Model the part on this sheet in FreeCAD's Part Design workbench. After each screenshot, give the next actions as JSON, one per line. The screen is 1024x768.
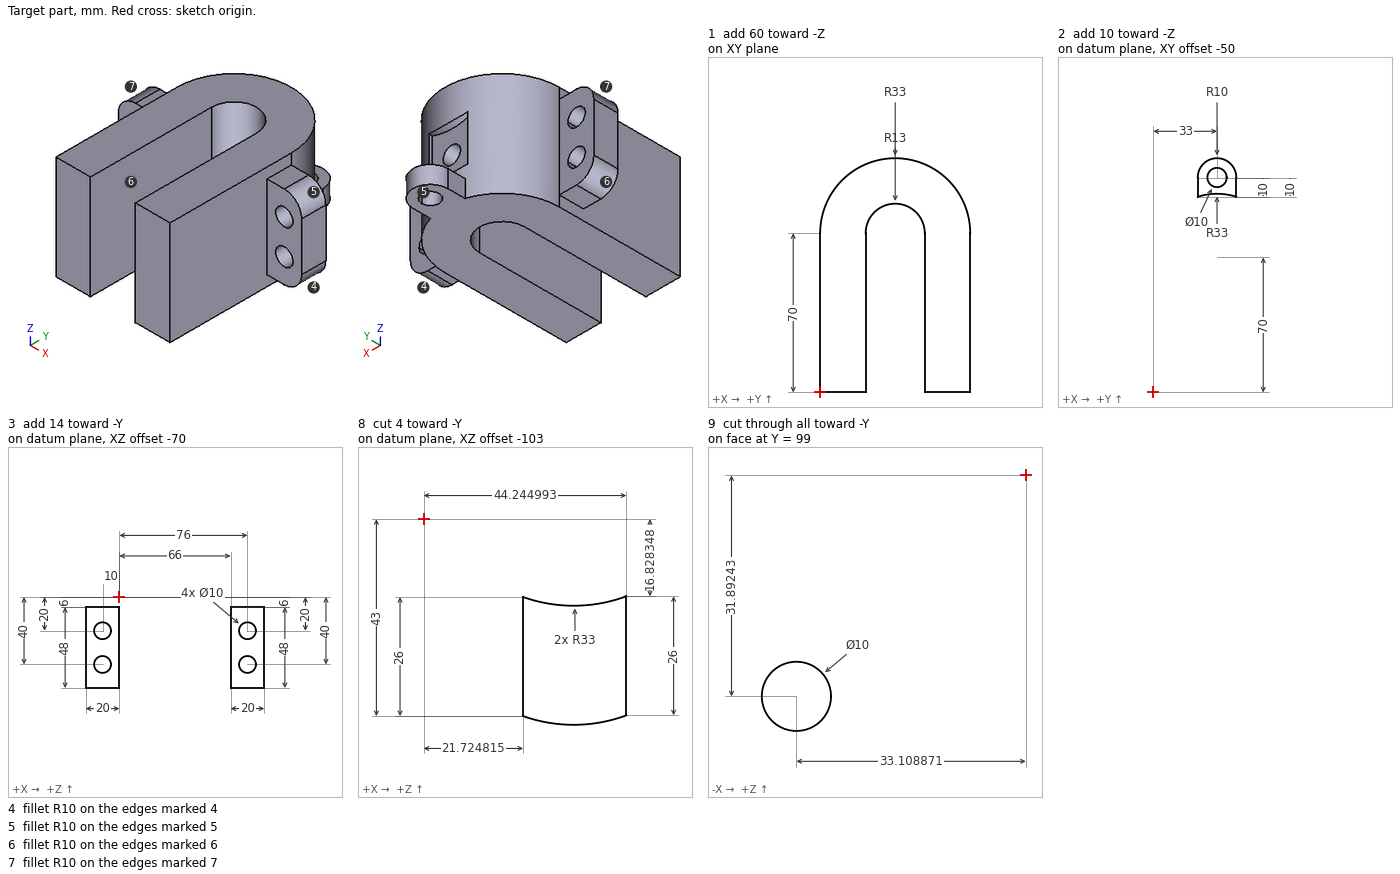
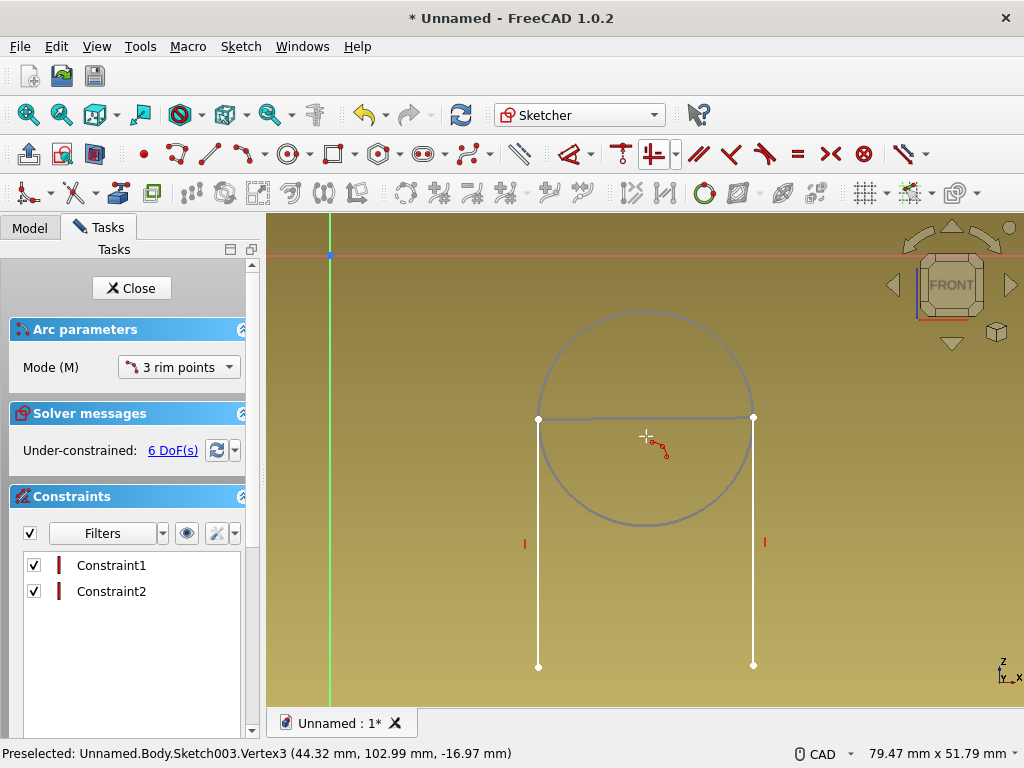
{"action": "left_click", "coordinate": [645, 436]}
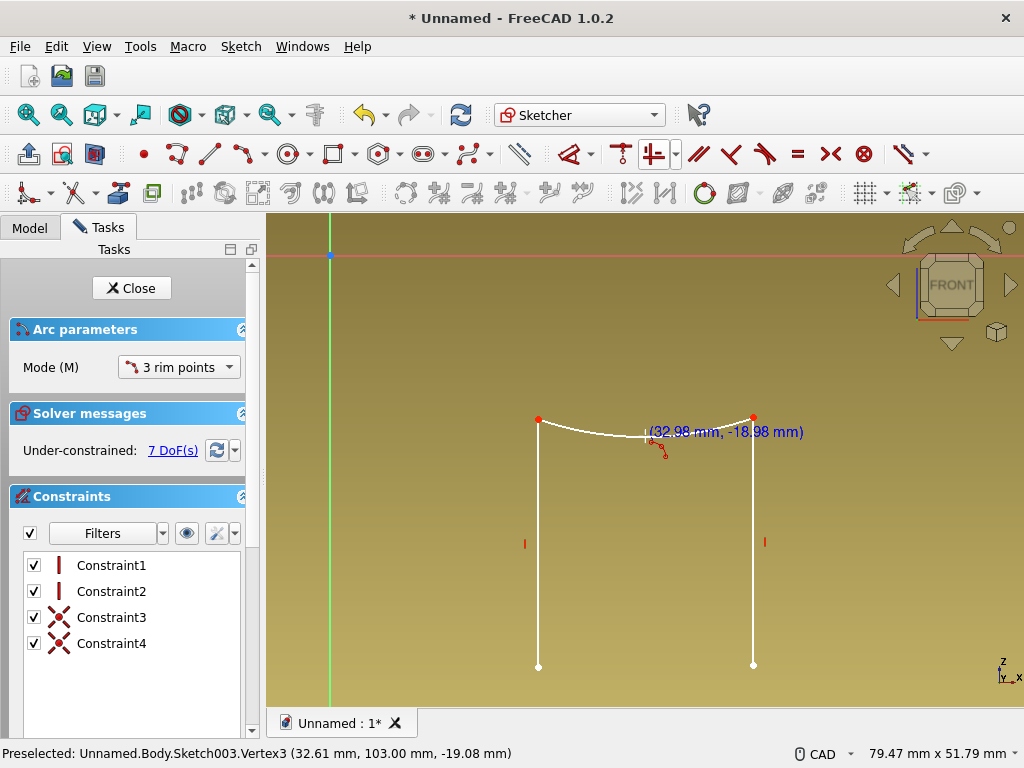
{"action": "left_click", "coordinate": [753, 666]}
{"action": "left_click", "coordinate": [538, 667]}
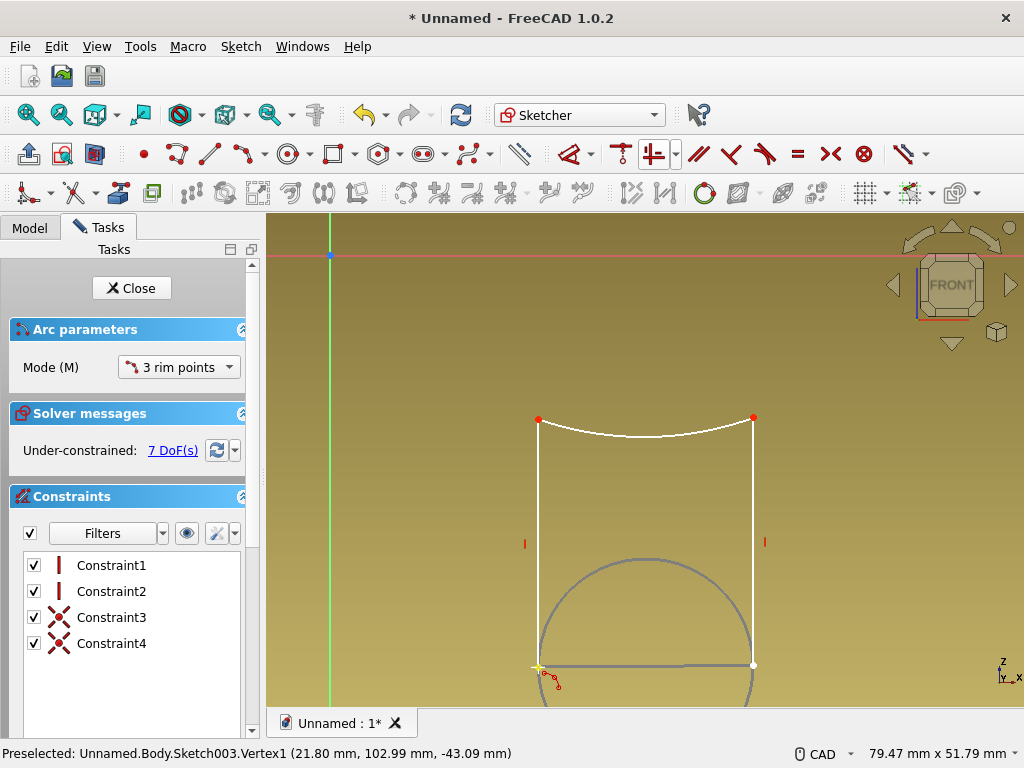
{"action": "scroll", "coordinate": [648, 440], "scroll_direction": "down", "scroll_amount": 2}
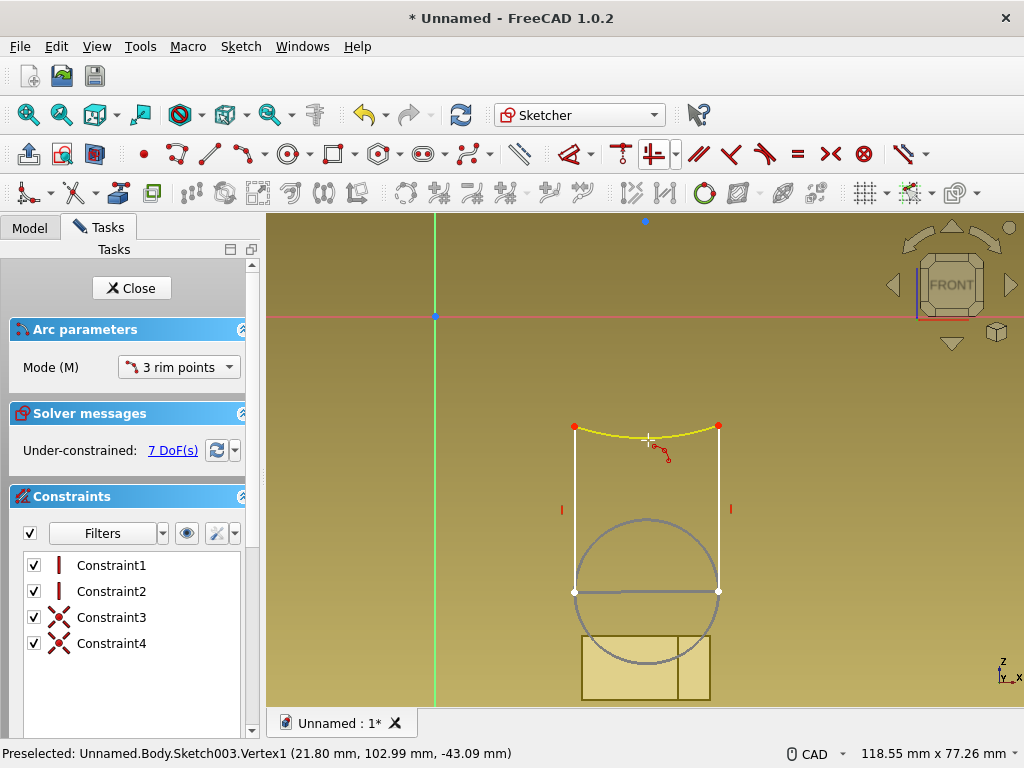
{"action": "scroll", "coordinate": [646, 604], "scroll_direction": "up", "scroll_amount": 2}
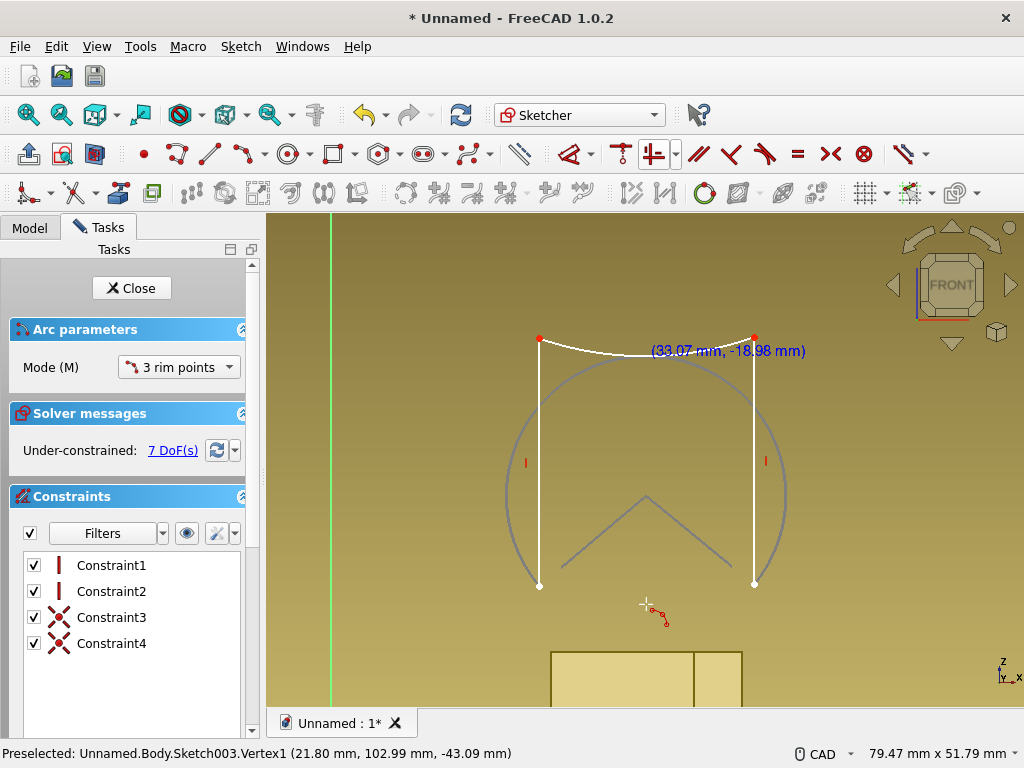
{"action": "left_click", "coordinate": [646, 603]}
{"action": "key", "text": "Escape"}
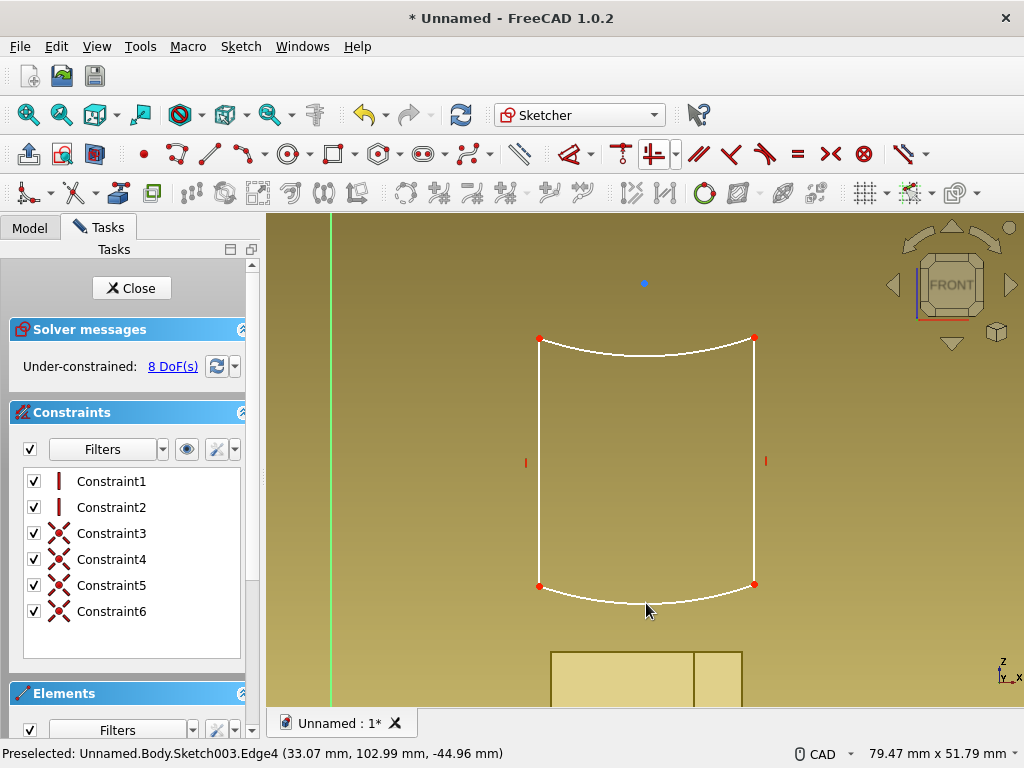
{"action": "left_click", "coordinate": [603, 354]}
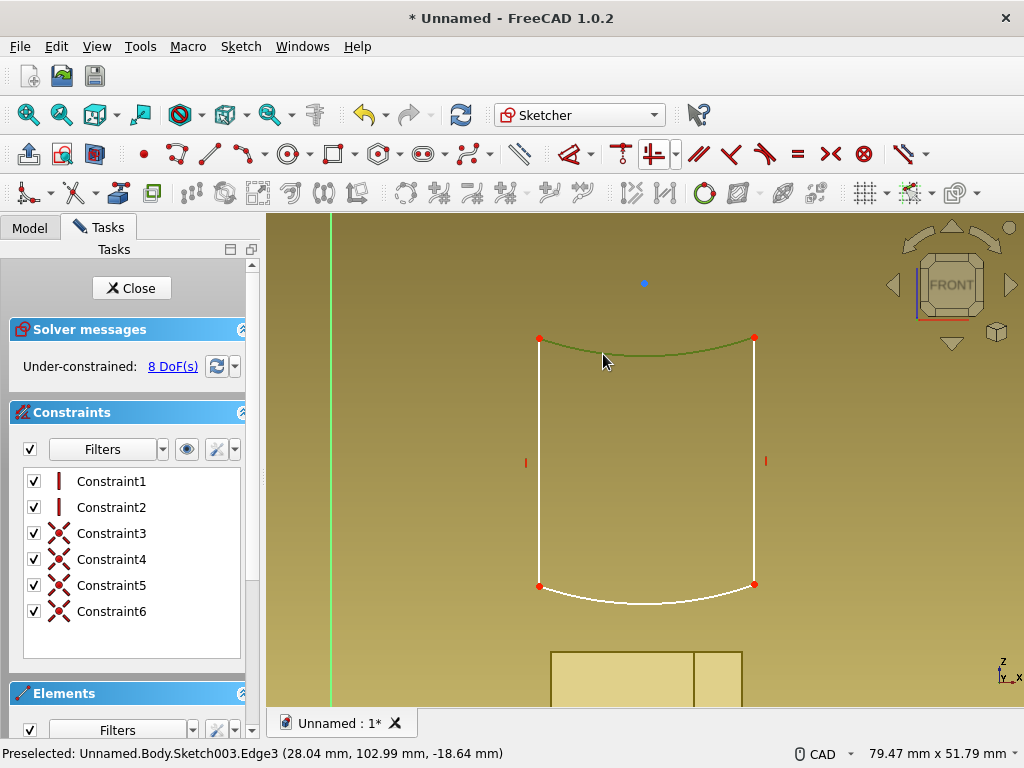
{"action": "left_click", "coordinate": [603, 601]}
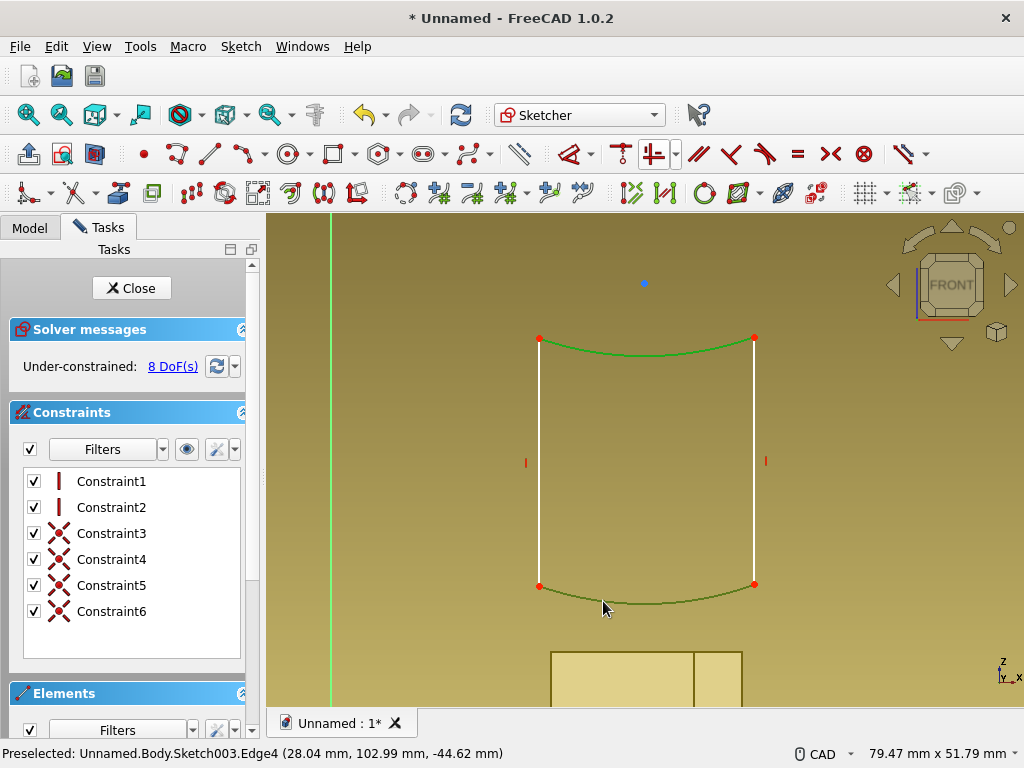
{"action": "left_click", "coordinate": [798, 154]}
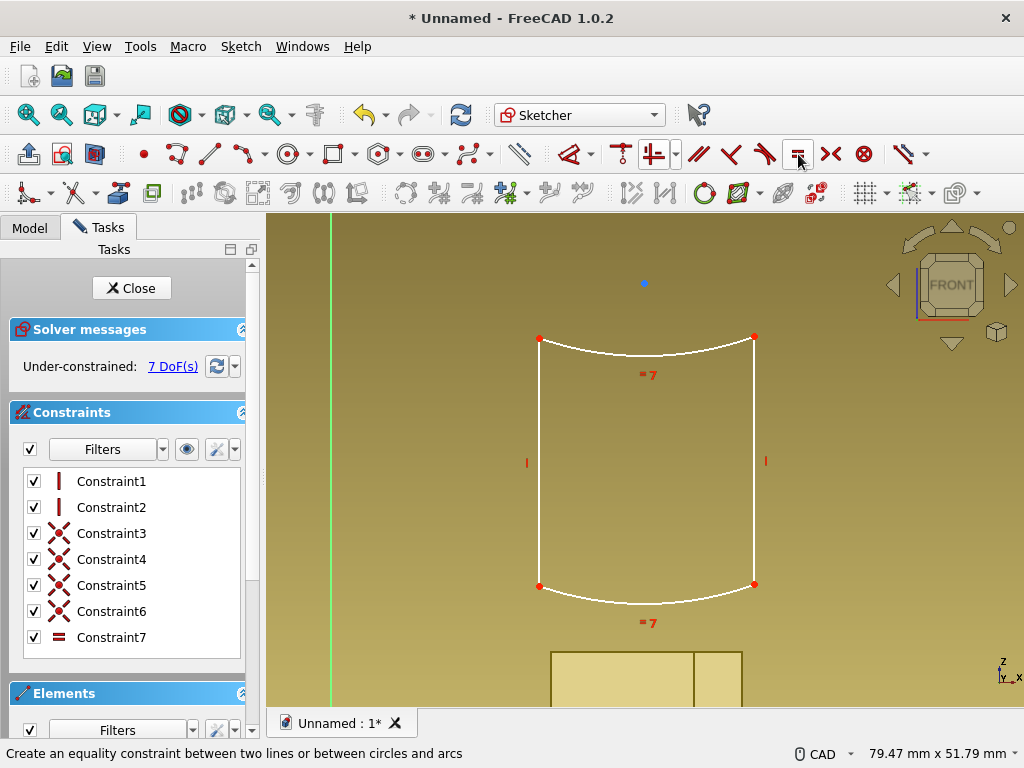
{"action": "key", "text": "d"}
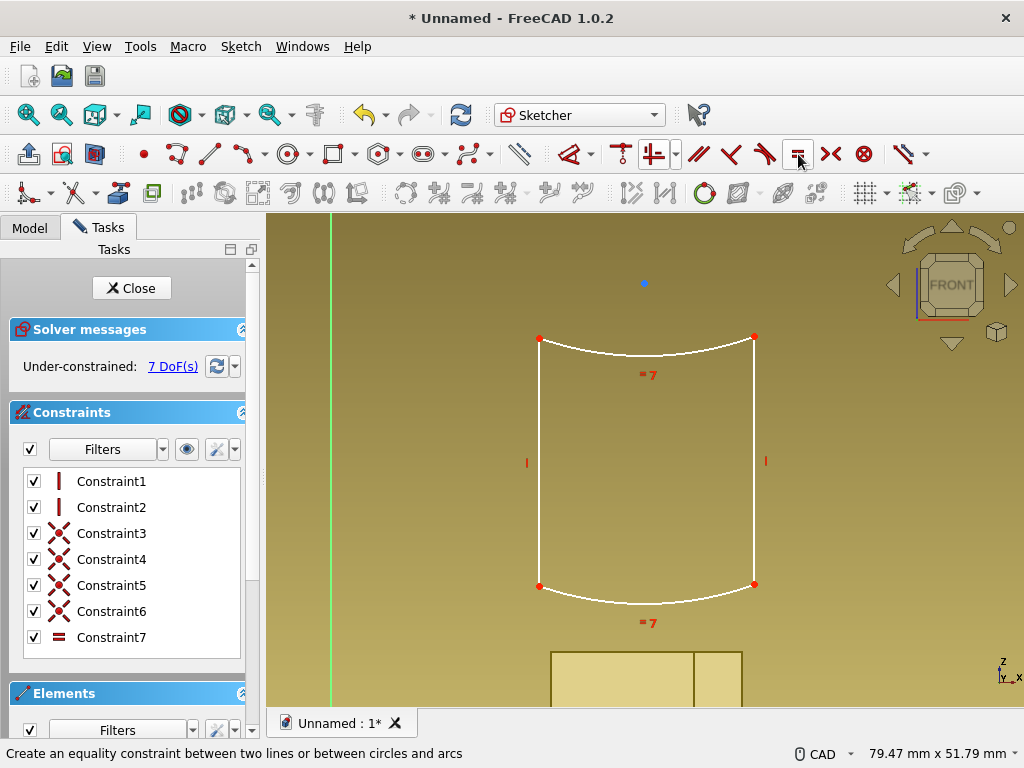
{"action": "left_click", "coordinate": [603, 353]}
{"action": "left_click", "coordinate": [599, 385]}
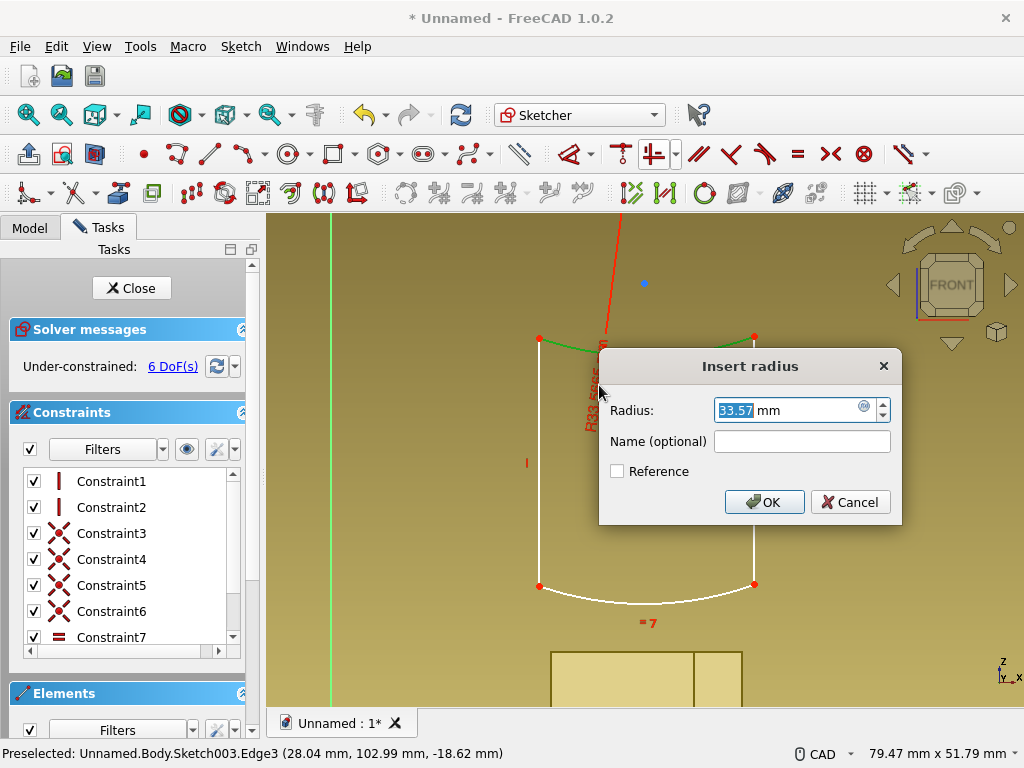
{"action": "type", "text": "33"}
{"action": "key", "text": "Return"}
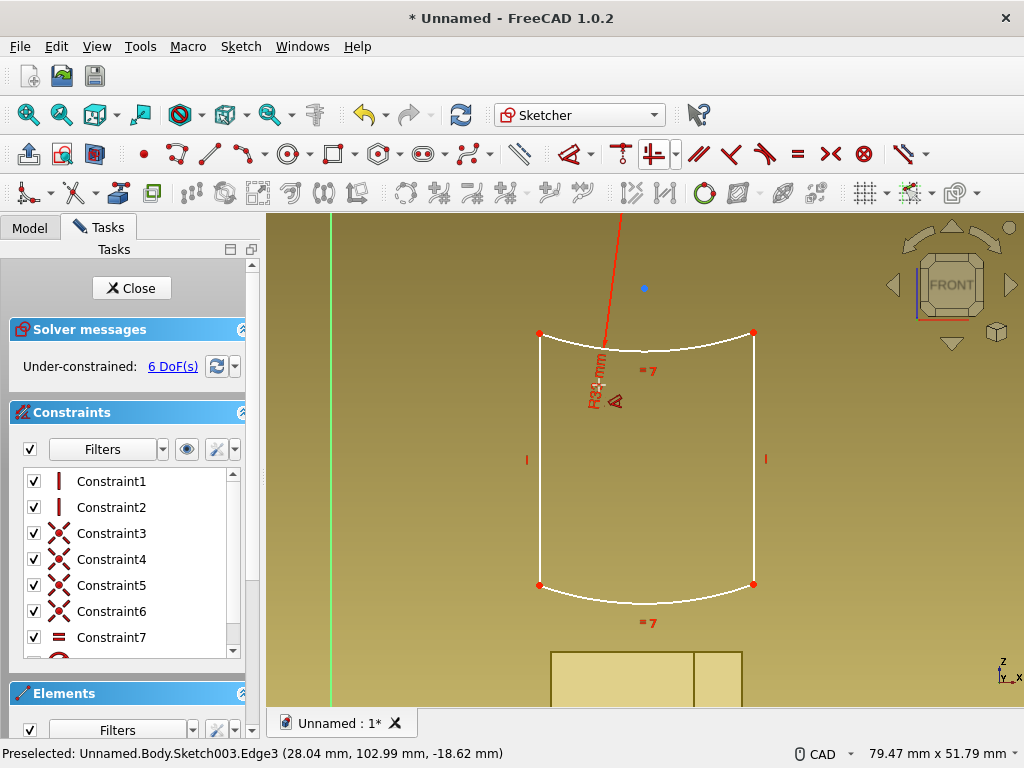
{"action": "left_click", "coordinate": [540, 510]}
{"action": "left_click", "coordinate": [506, 460]}